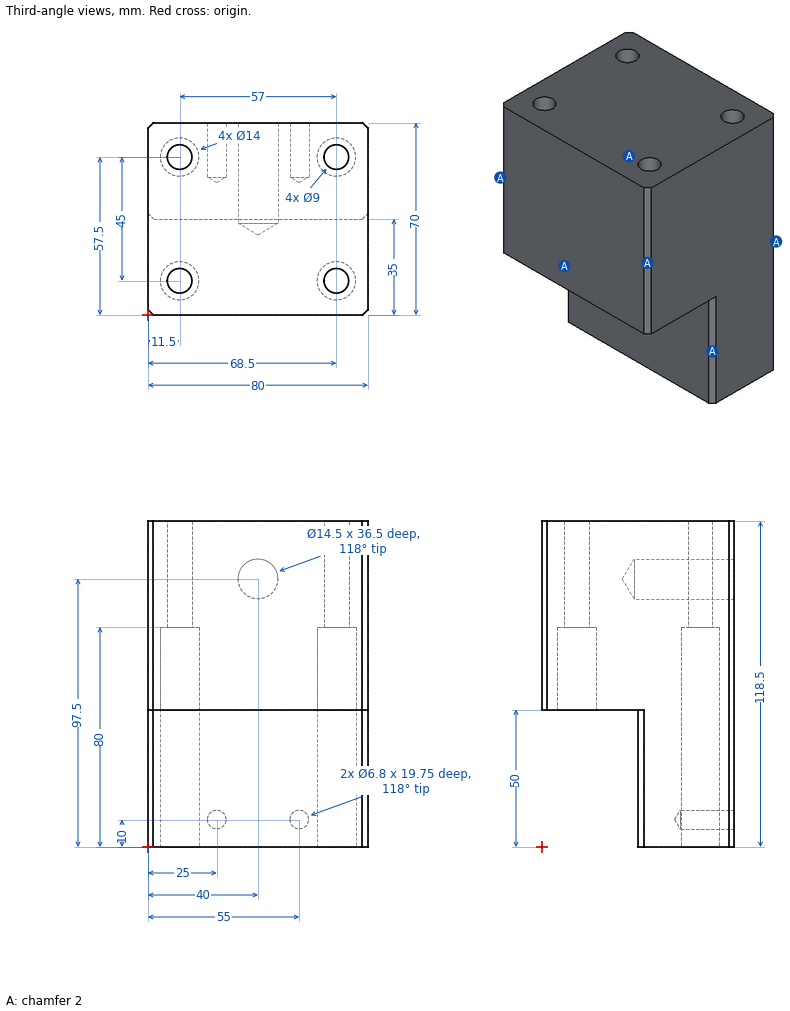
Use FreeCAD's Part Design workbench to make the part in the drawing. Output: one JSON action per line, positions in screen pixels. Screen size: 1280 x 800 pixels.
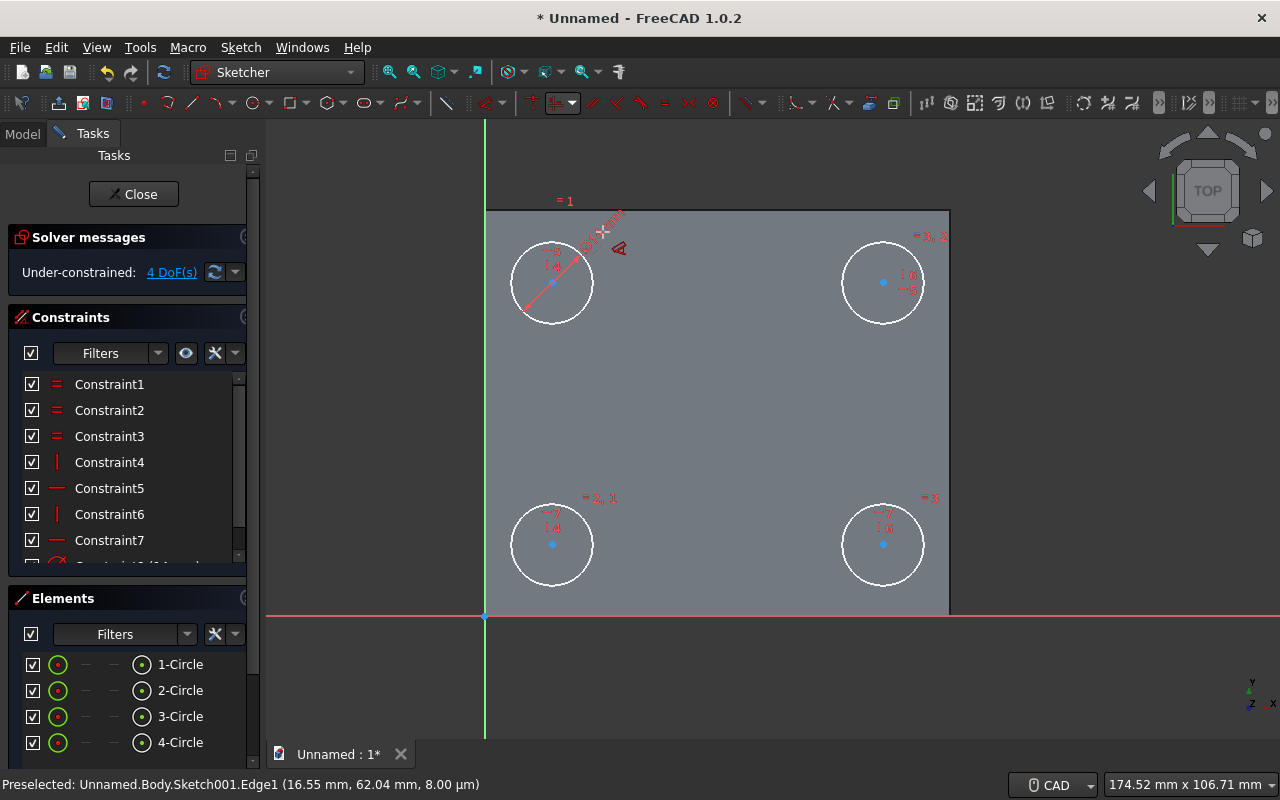
{"action": "left_click", "coordinate": [552, 283]}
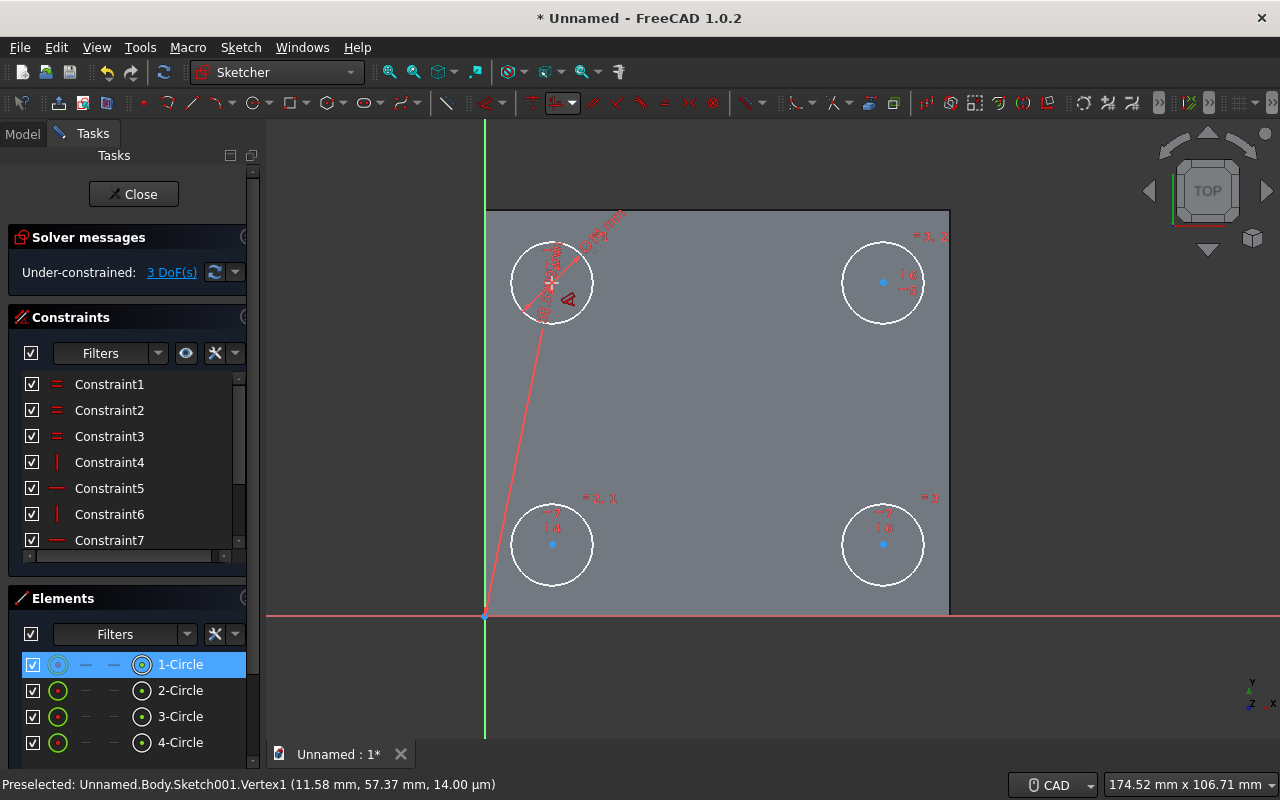
{"action": "left_click", "coordinate": [552, 545]}
{"action": "left_click", "coordinate": [518, 414]}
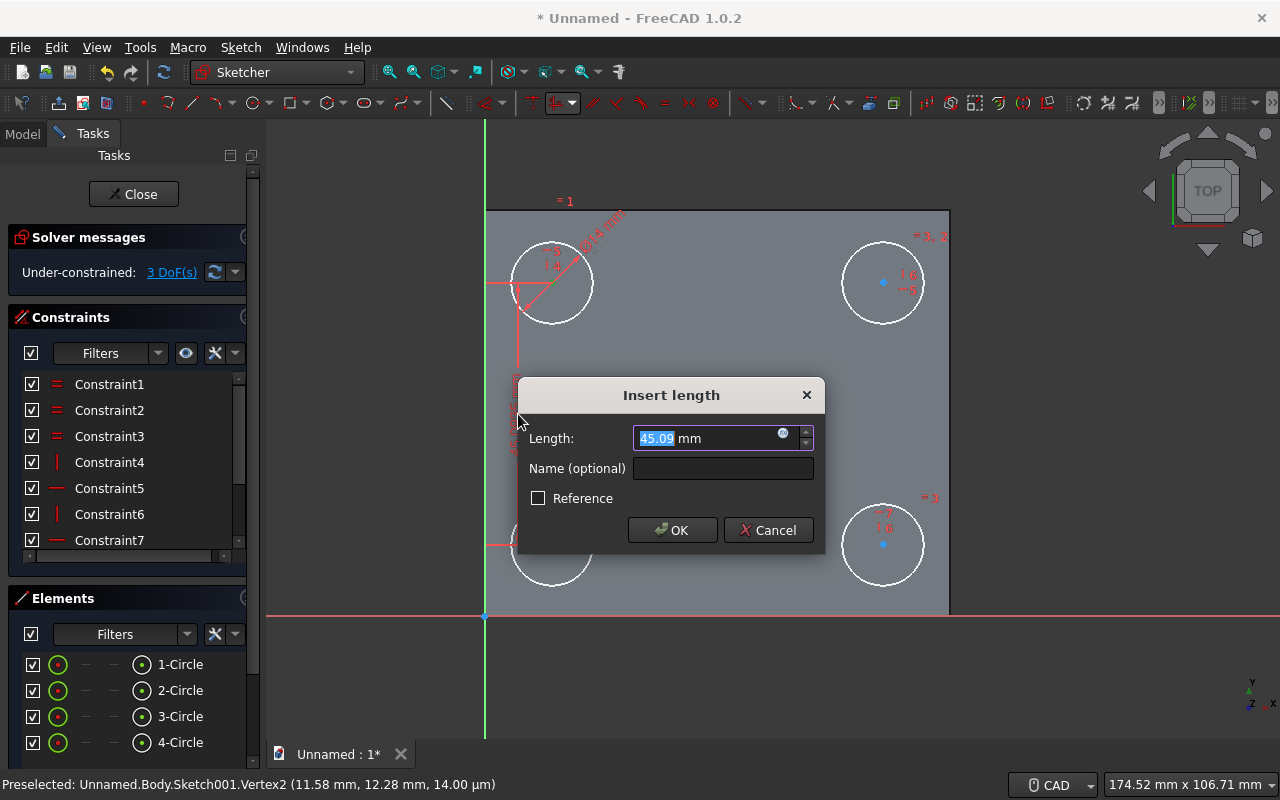
{"action": "type", "text": "45"}
{"action": "key", "text": "Return"}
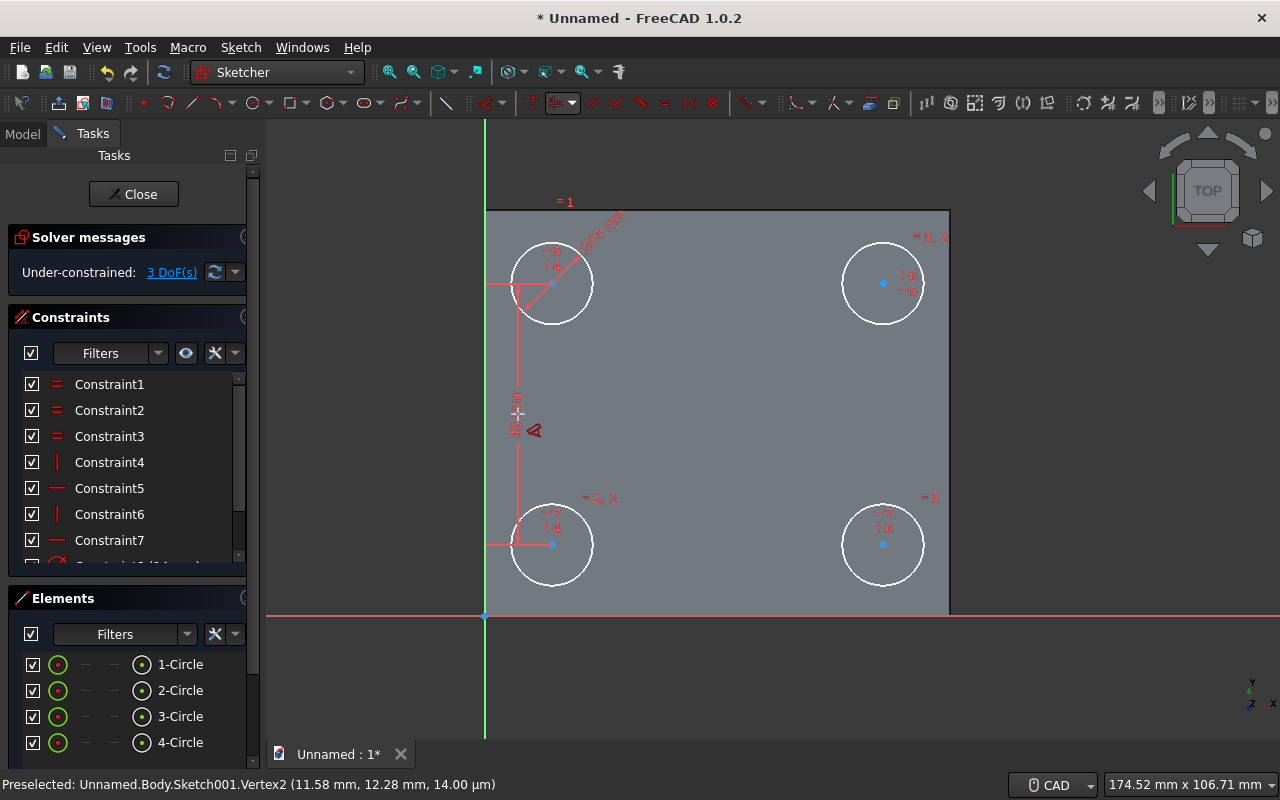
{"action": "left_click", "coordinate": [552, 284]}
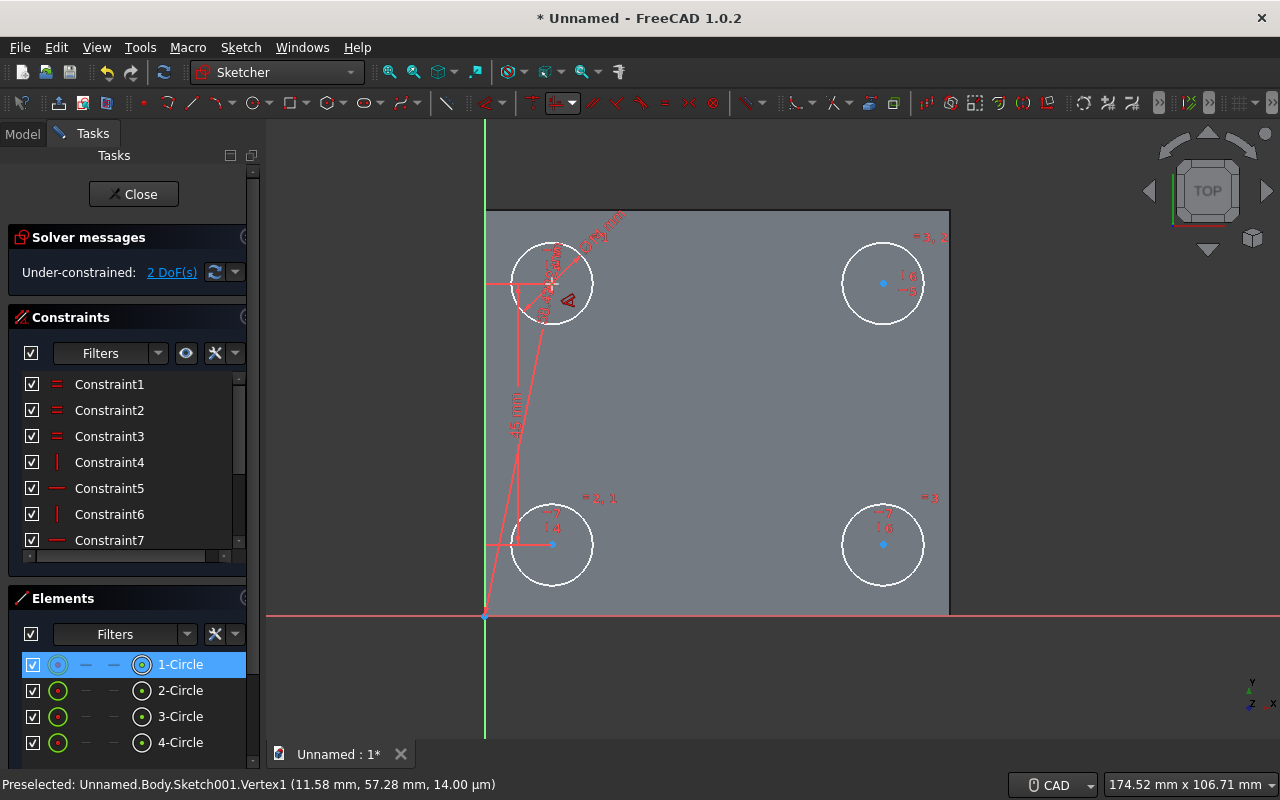
{"action": "left_click", "coordinate": [883, 284]}
{"action": "left_click", "coordinate": [718, 250]}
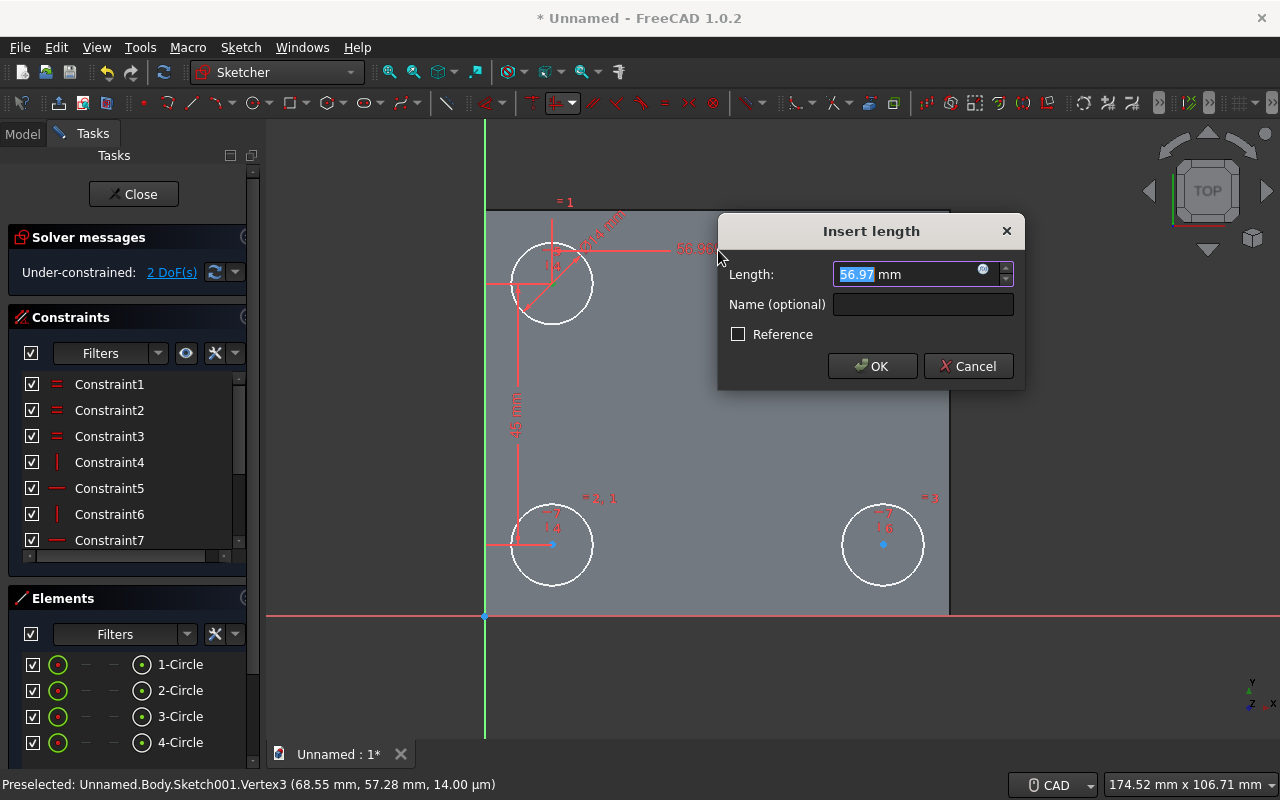
{"action": "type", "text": "57"}
{"action": "key", "text": "Return"}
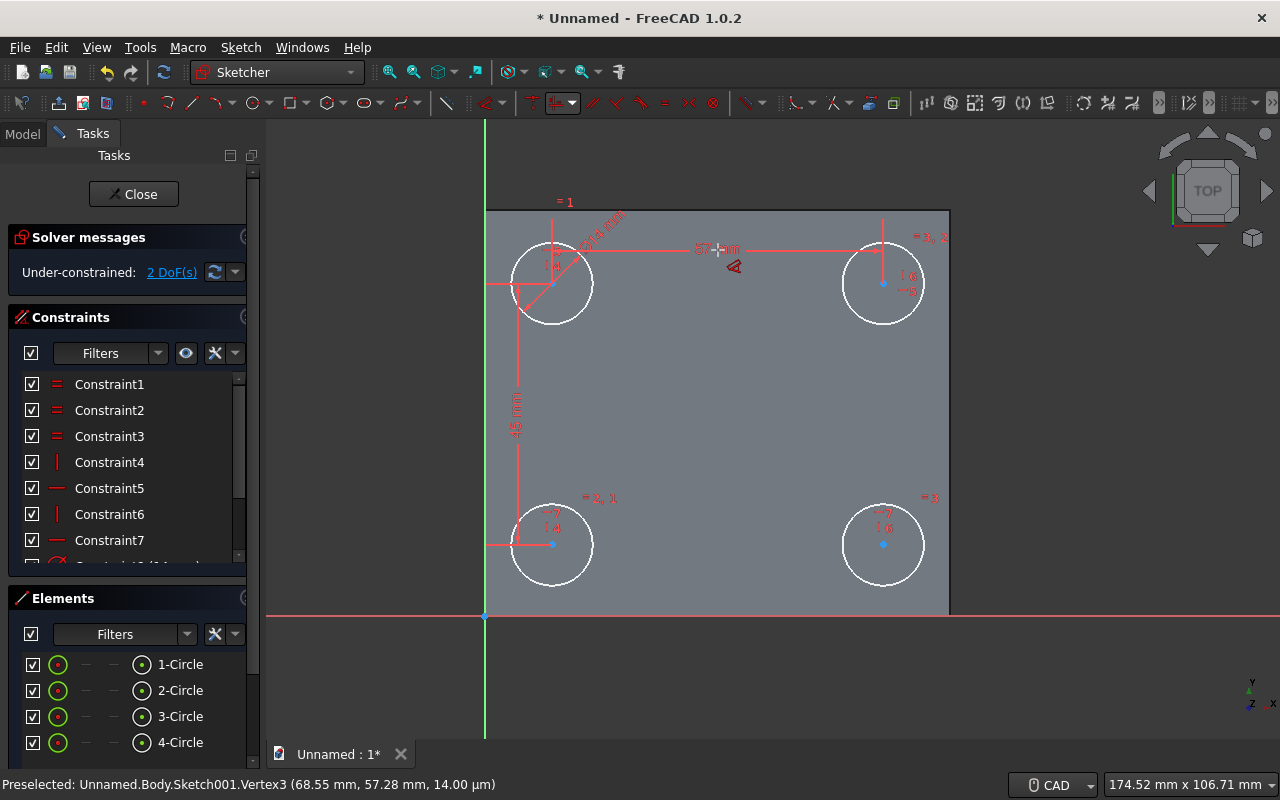
{"action": "left_click", "coordinate": [552, 284]}
{"action": "left_click", "coordinate": [518, 650]}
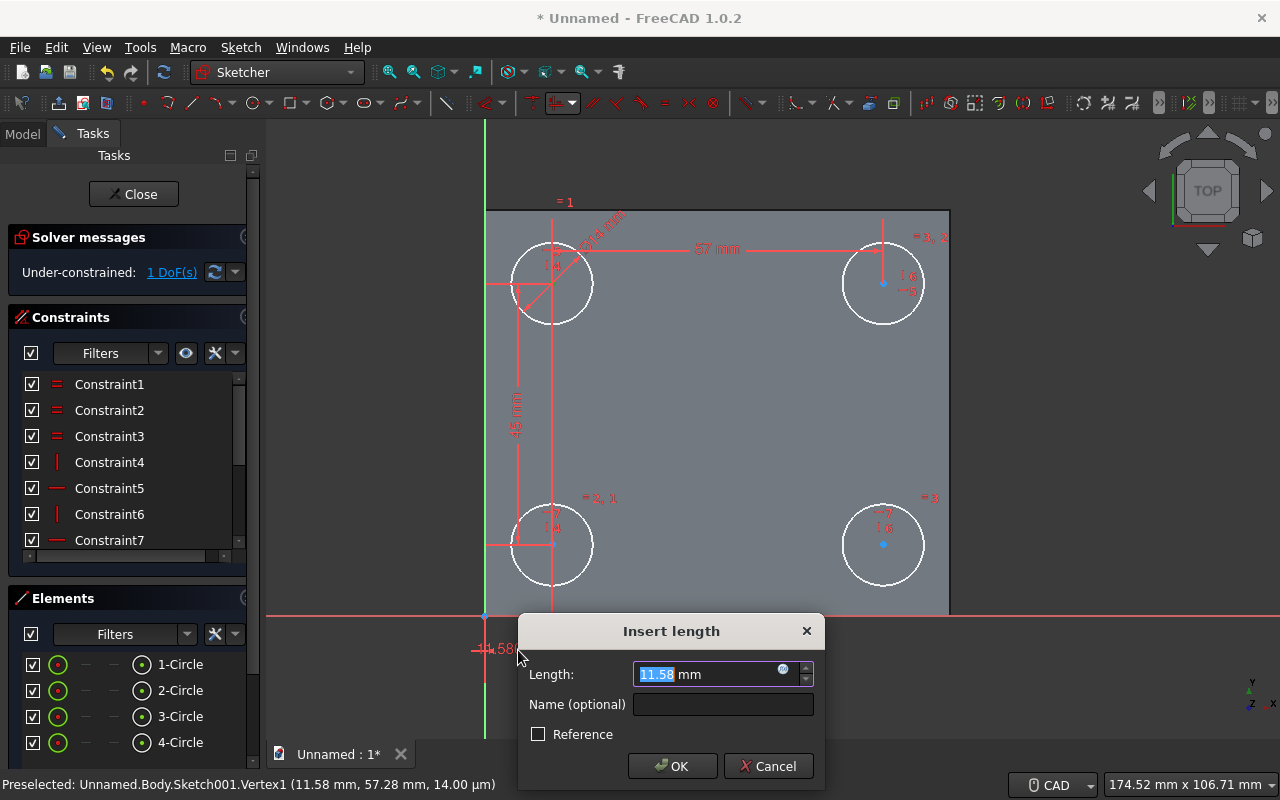
{"action": "type", "text": "11.5"}
{"action": "key", "text": "Return"}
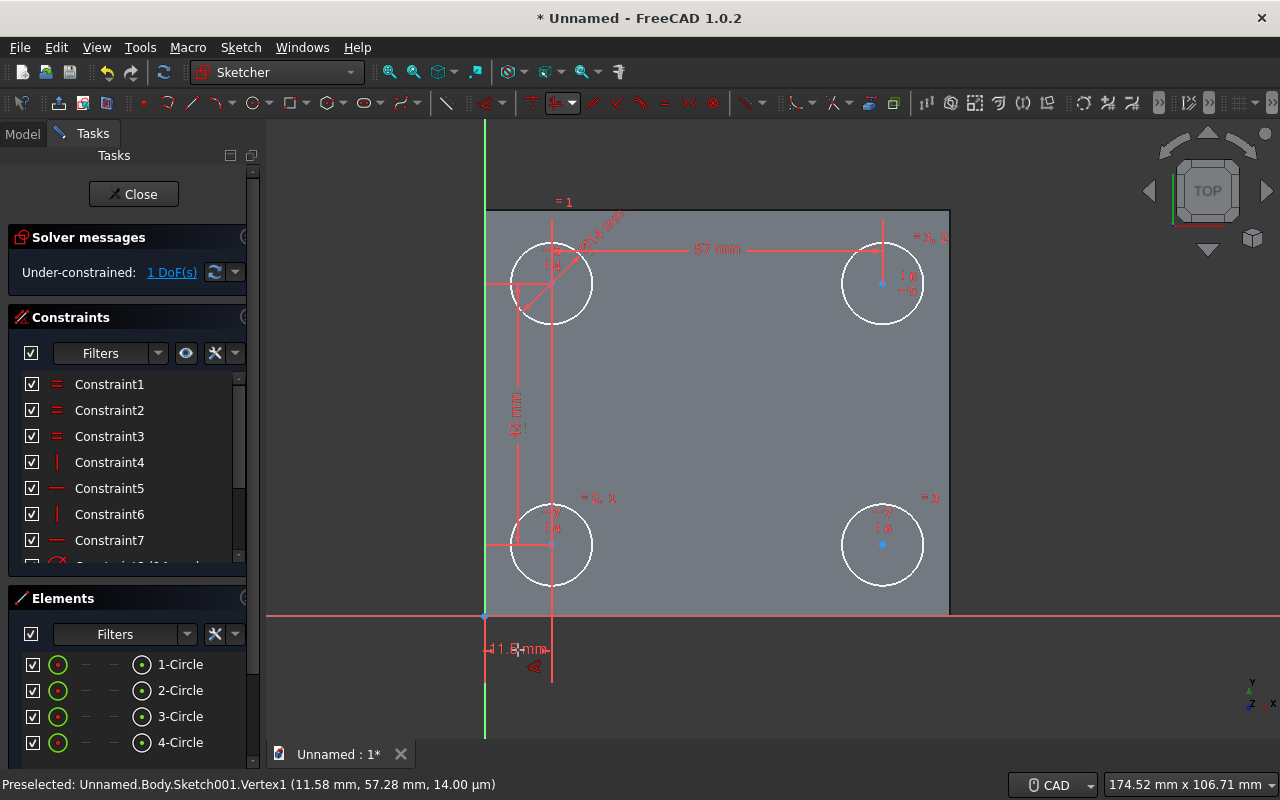
{"action": "left_click", "coordinate": [552, 284]}
{"action": "left_click", "coordinate": [451, 450]}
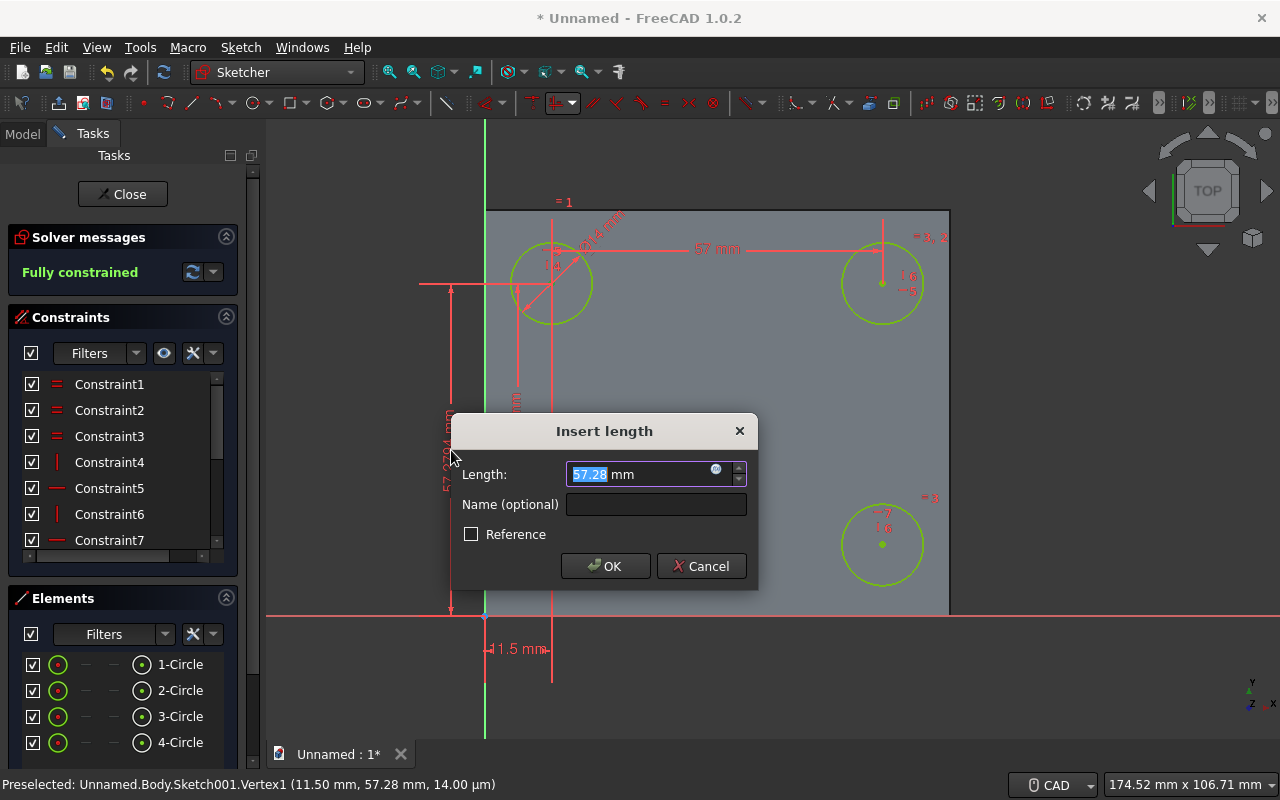
{"action": "type", "text": "57.5"}
{"action": "key", "text": "Return"}
{"action": "key", "text": "Escape"}